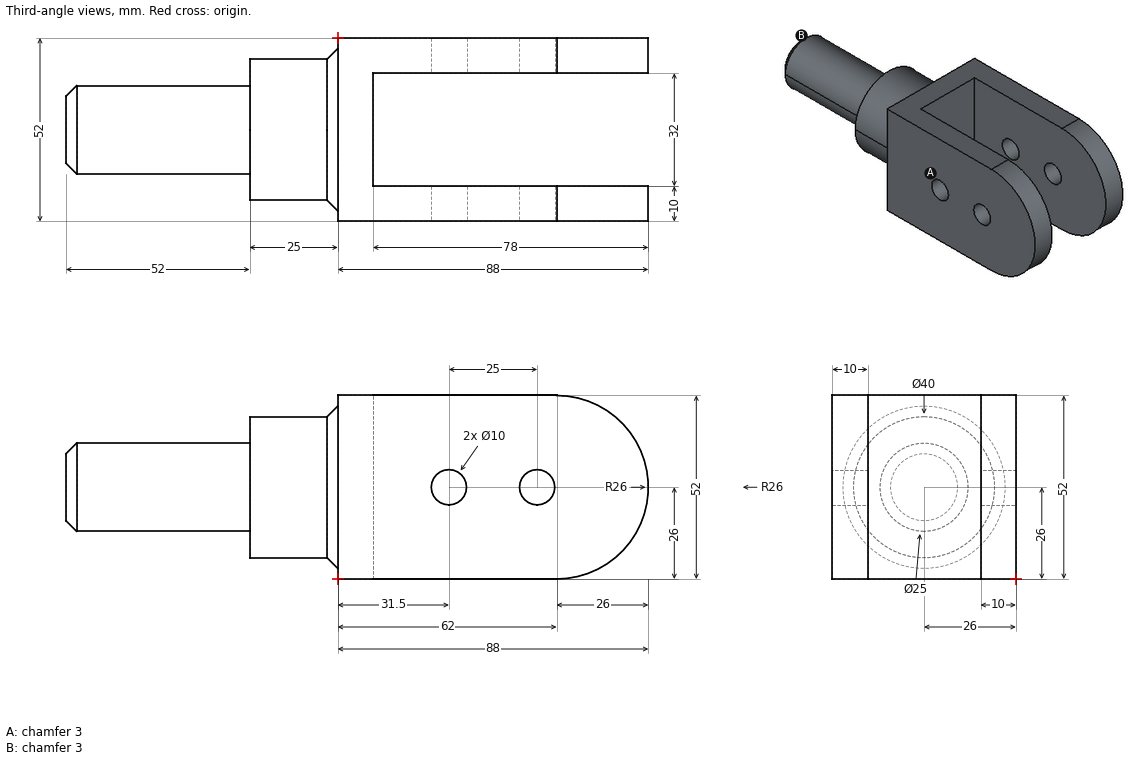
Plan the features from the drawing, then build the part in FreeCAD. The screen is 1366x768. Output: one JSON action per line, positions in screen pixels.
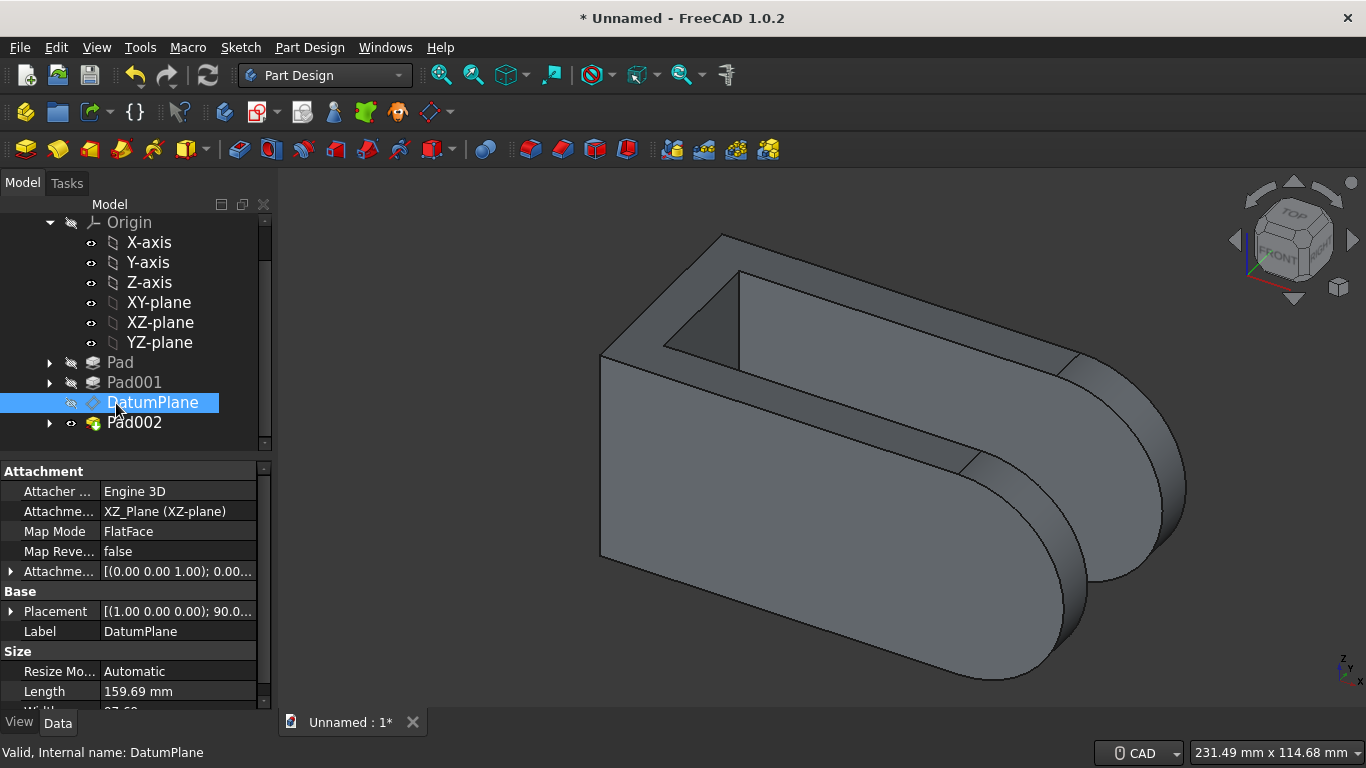
{"action": "left_click", "coordinate": [442, 76]}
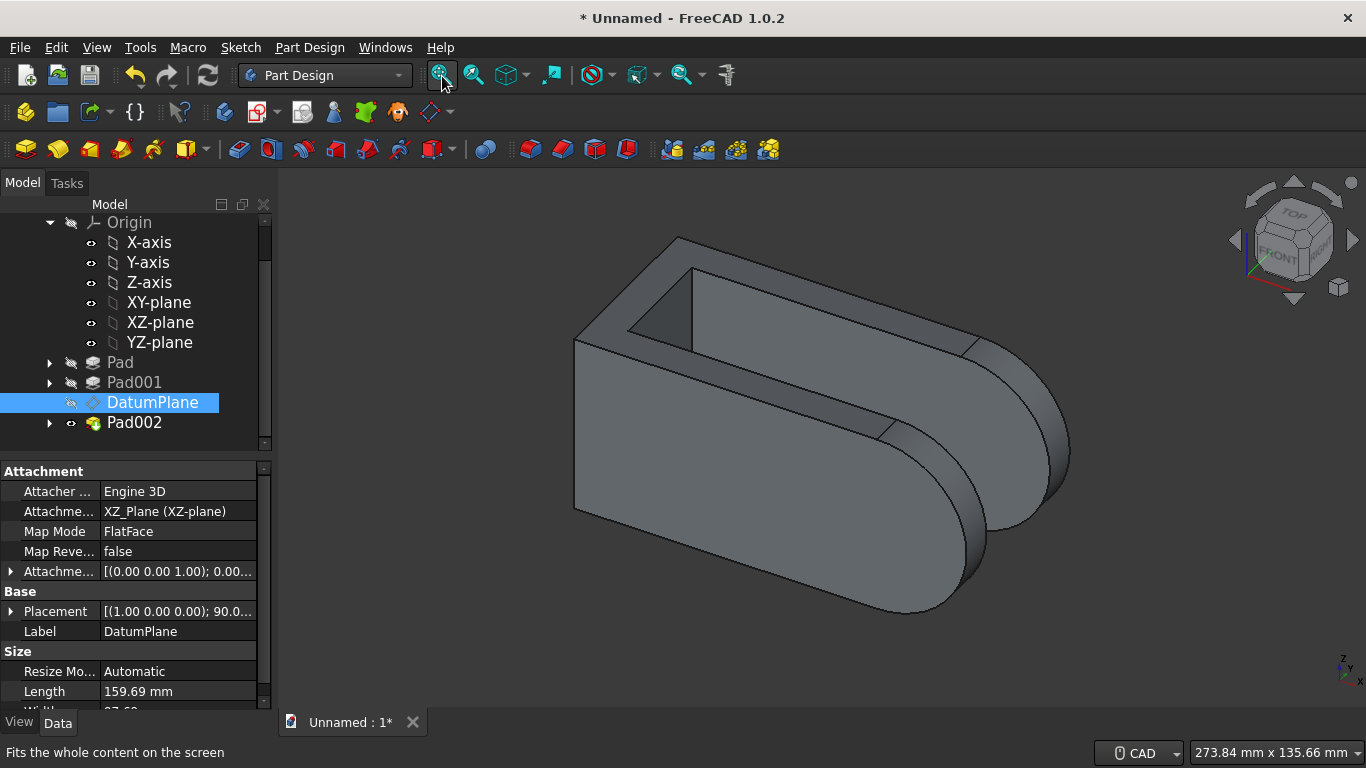
{"action": "left_click", "coordinate": [136, 323]}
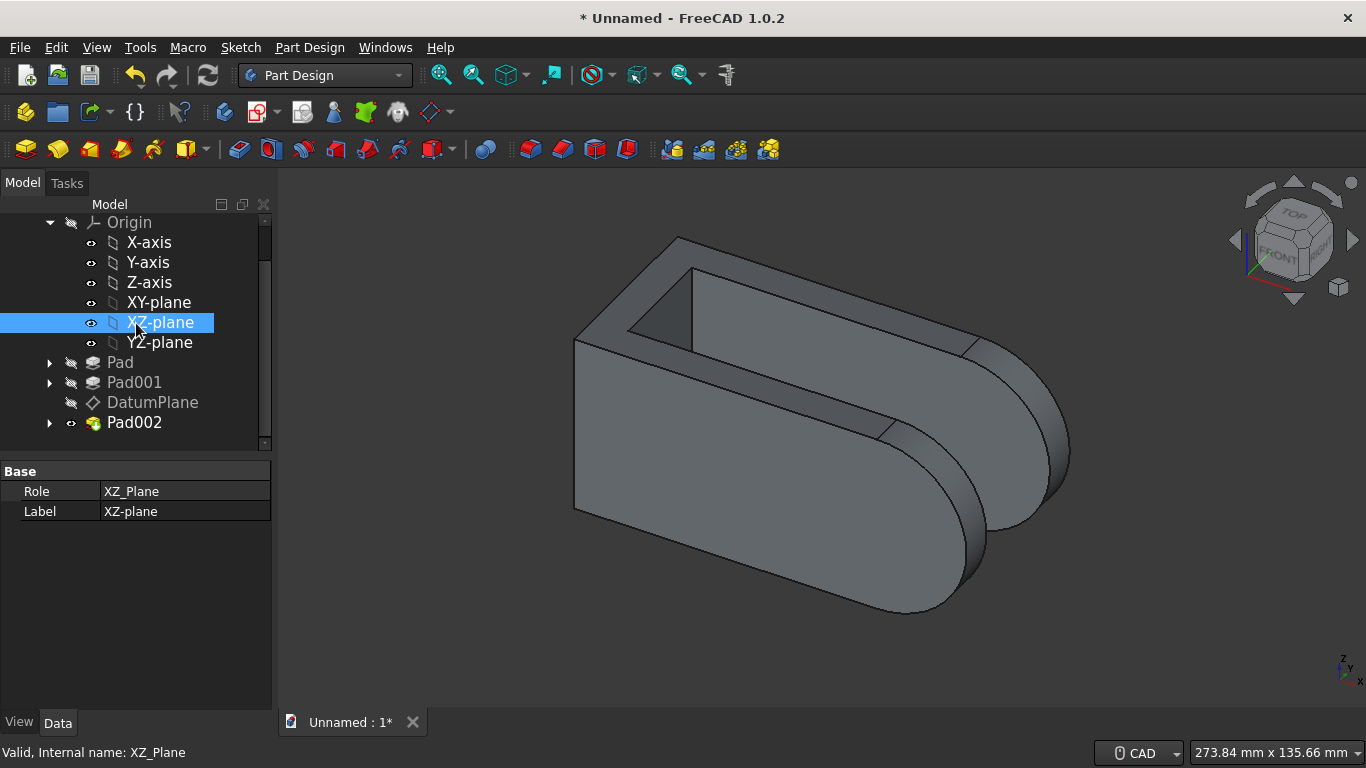
{"action": "left_click", "coordinate": [430, 112]}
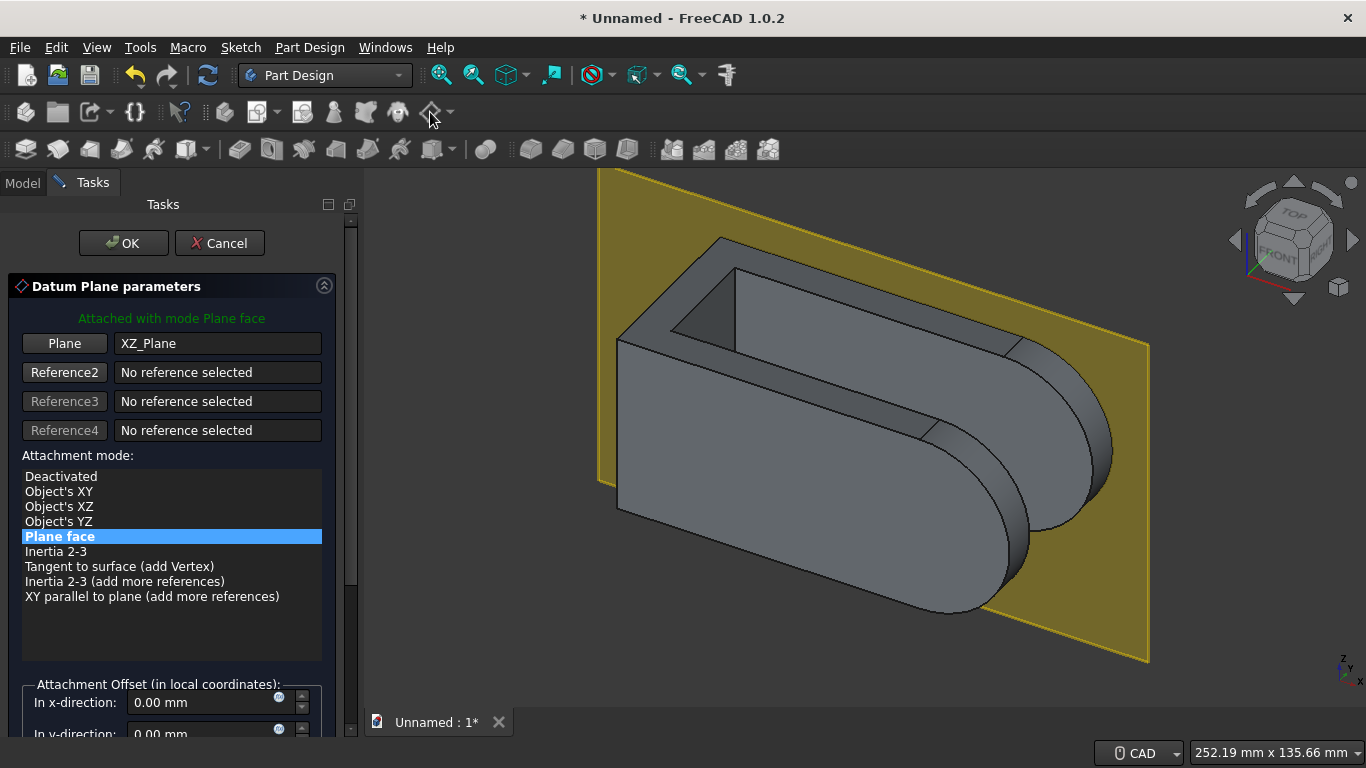
{"action": "scroll", "coordinate": [351, 475], "scroll_direction": "down", "scroll_amount": 2}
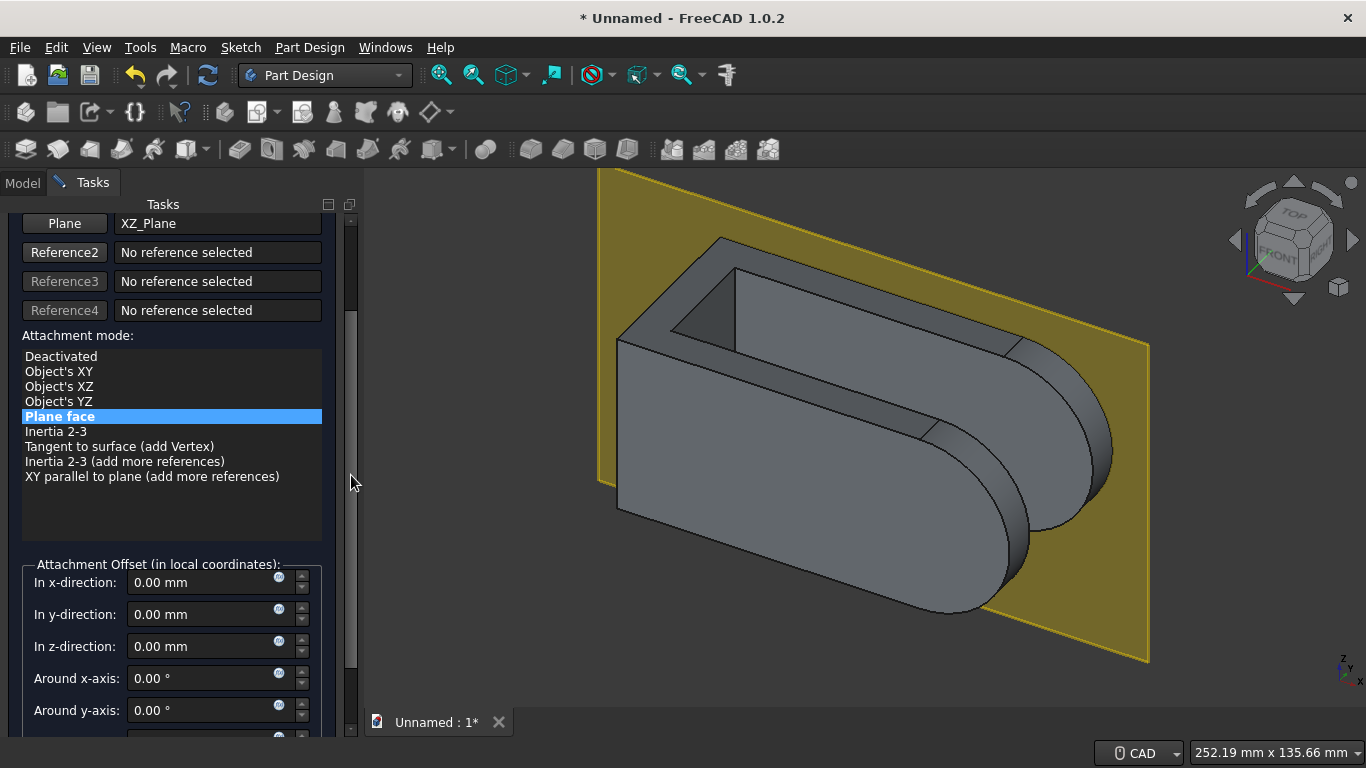
{"action": "triple_click", "coordinate": [210, 646]}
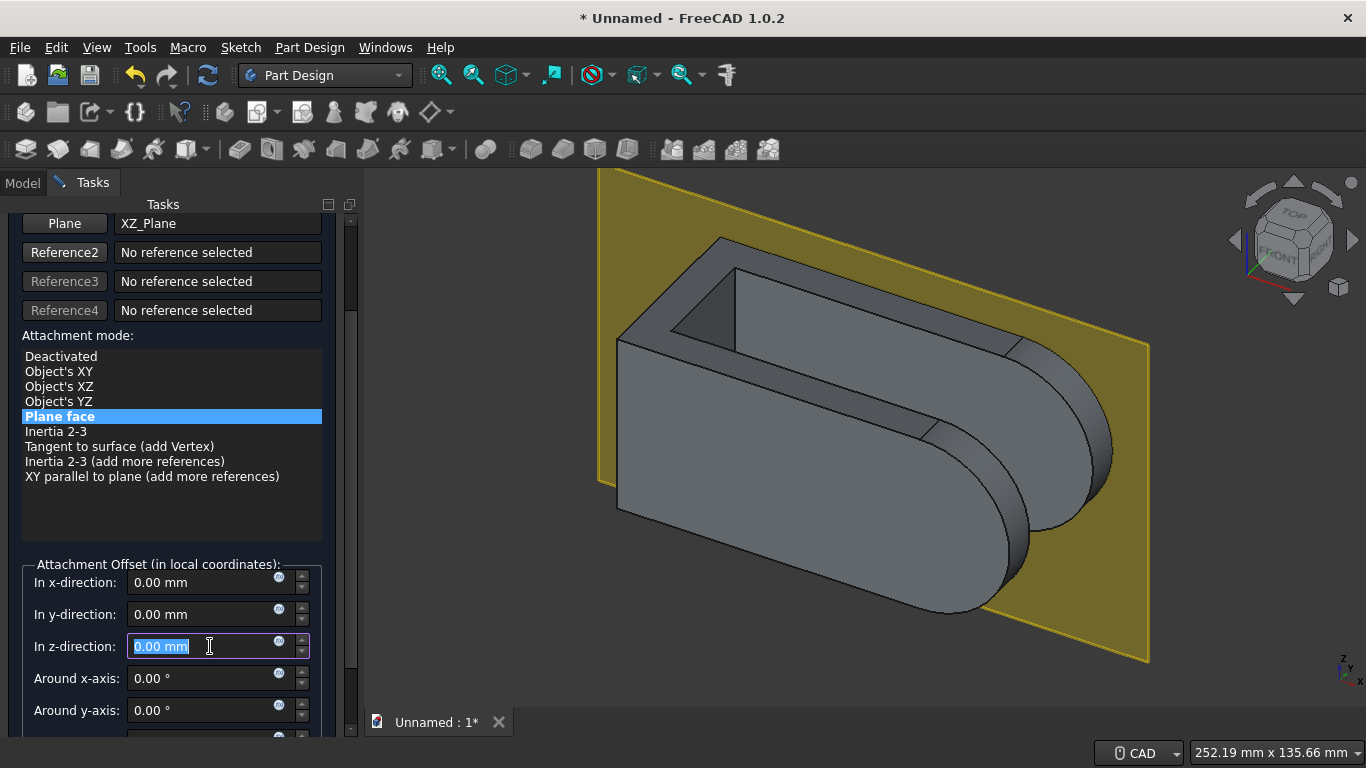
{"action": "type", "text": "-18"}
{"action": "key", "text": "Tab"}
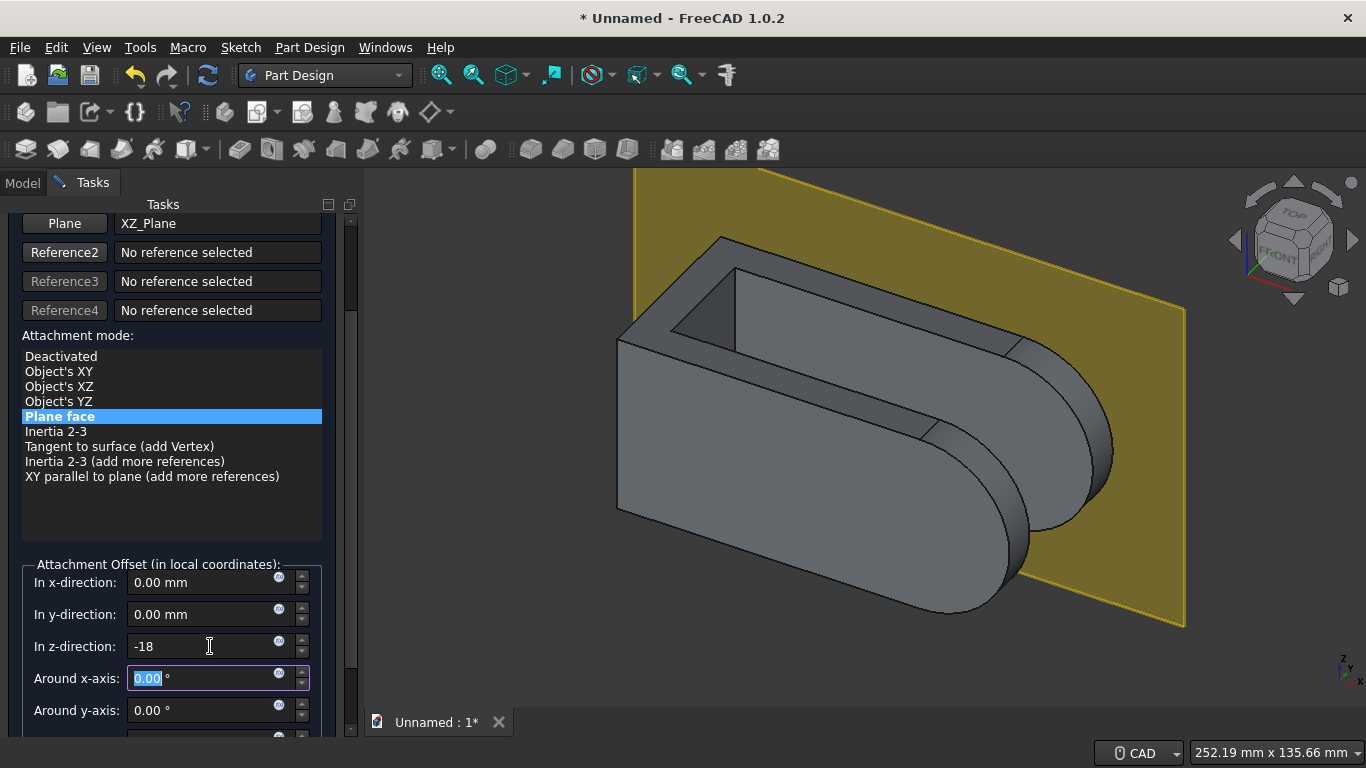
{"action": "scroll", "coordinate": [351, 475], "scroll_direction": "up", "scroll_amount": 3}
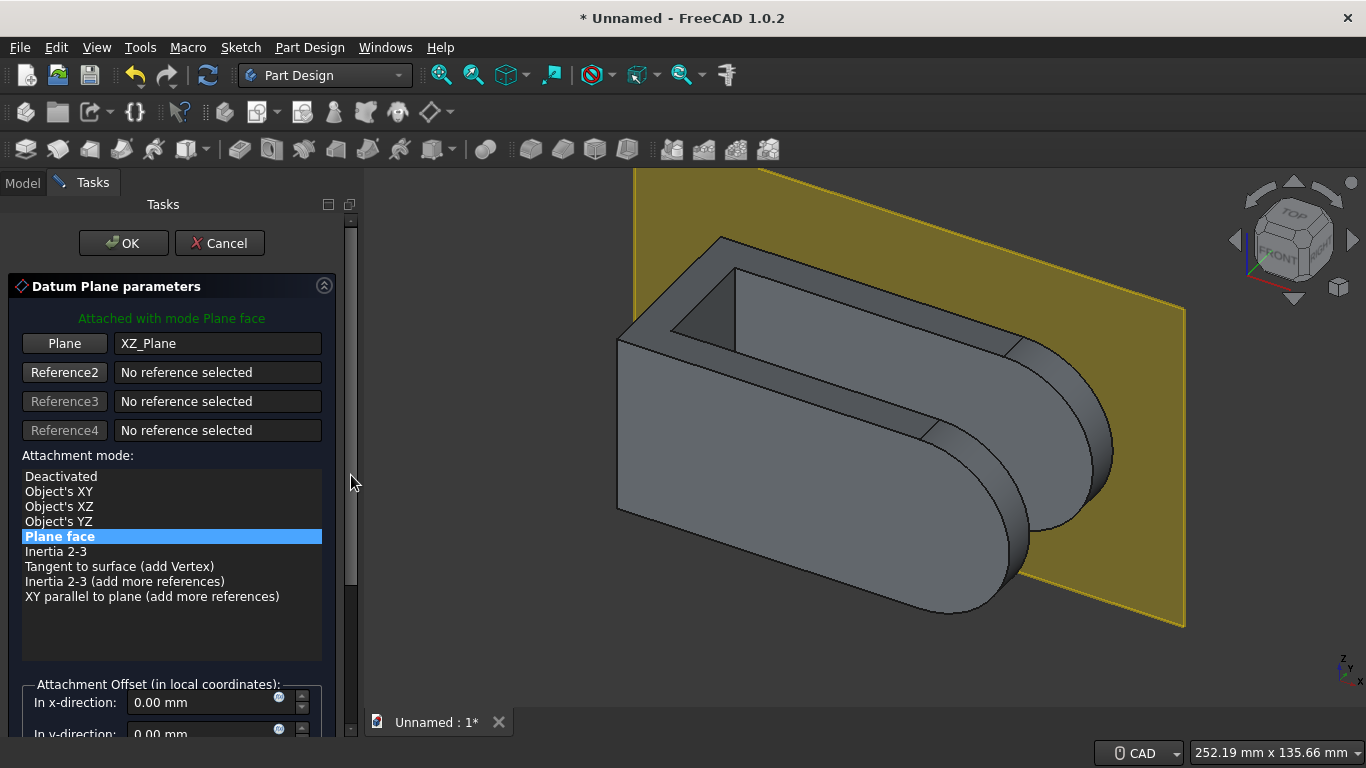
{"action": "left_click", "coordinate": [124, 243]}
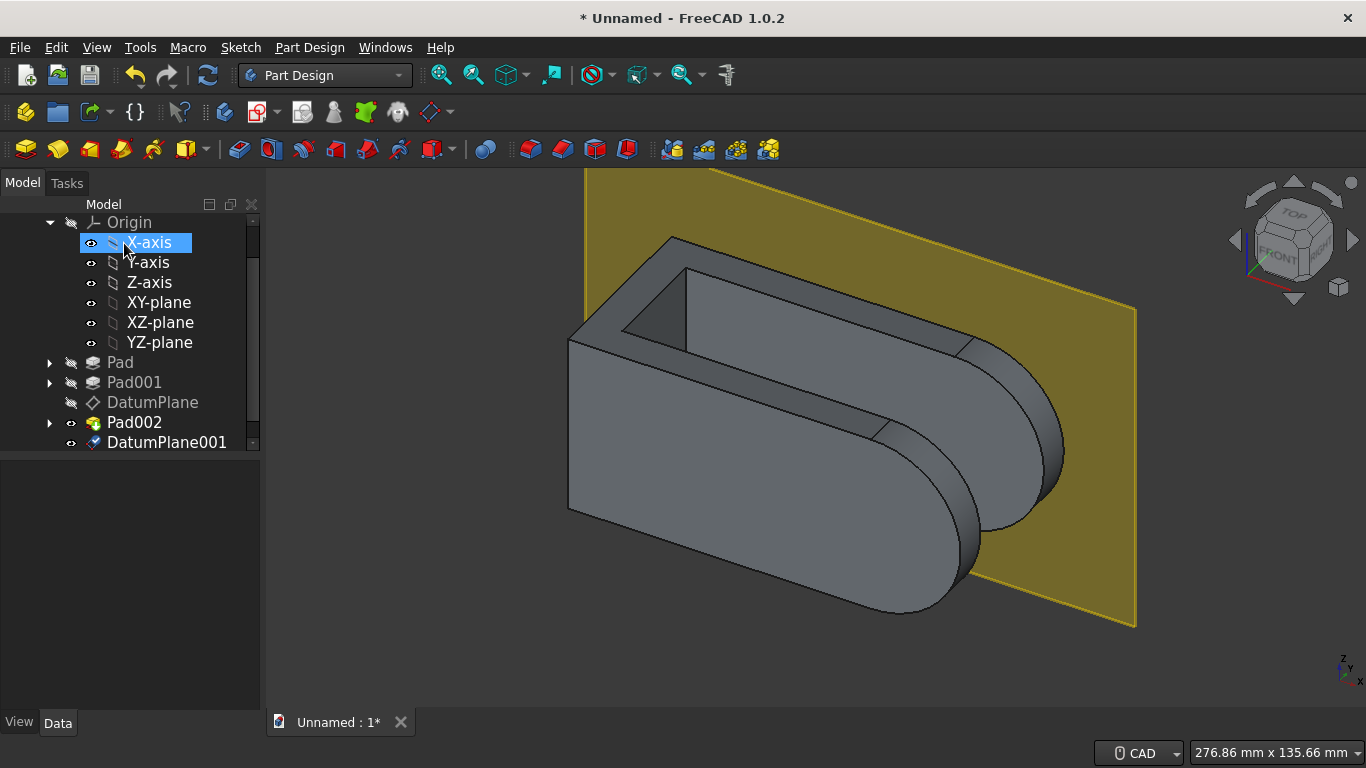
{"action": "left_click", "coordinate": [116, 443]}